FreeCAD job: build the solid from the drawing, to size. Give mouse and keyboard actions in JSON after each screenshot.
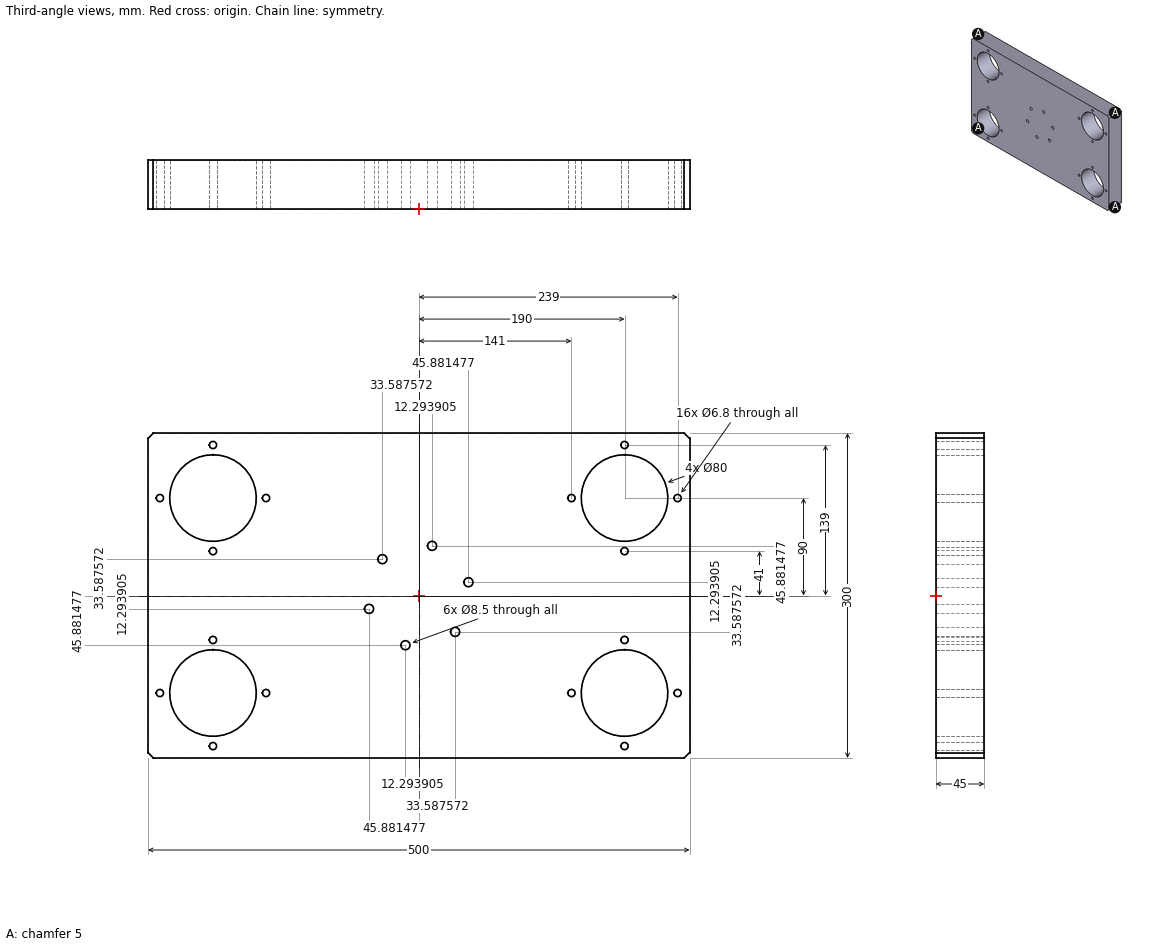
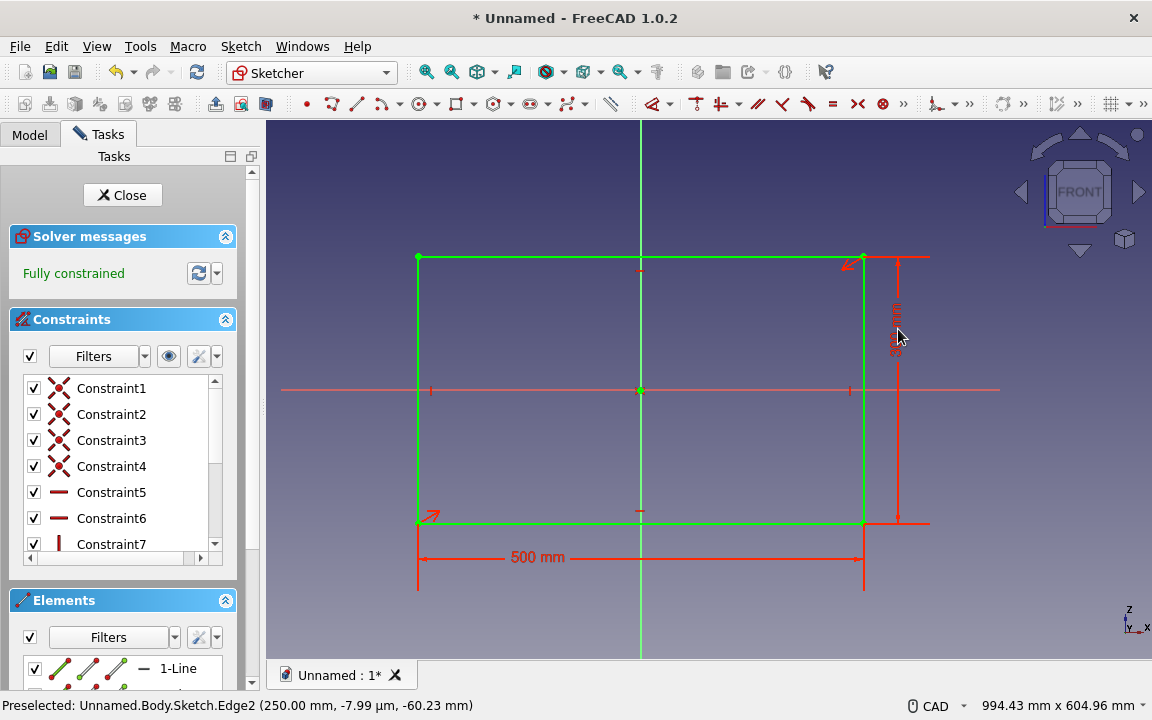
{"action": "left_click", "coordinate": [123, 195]}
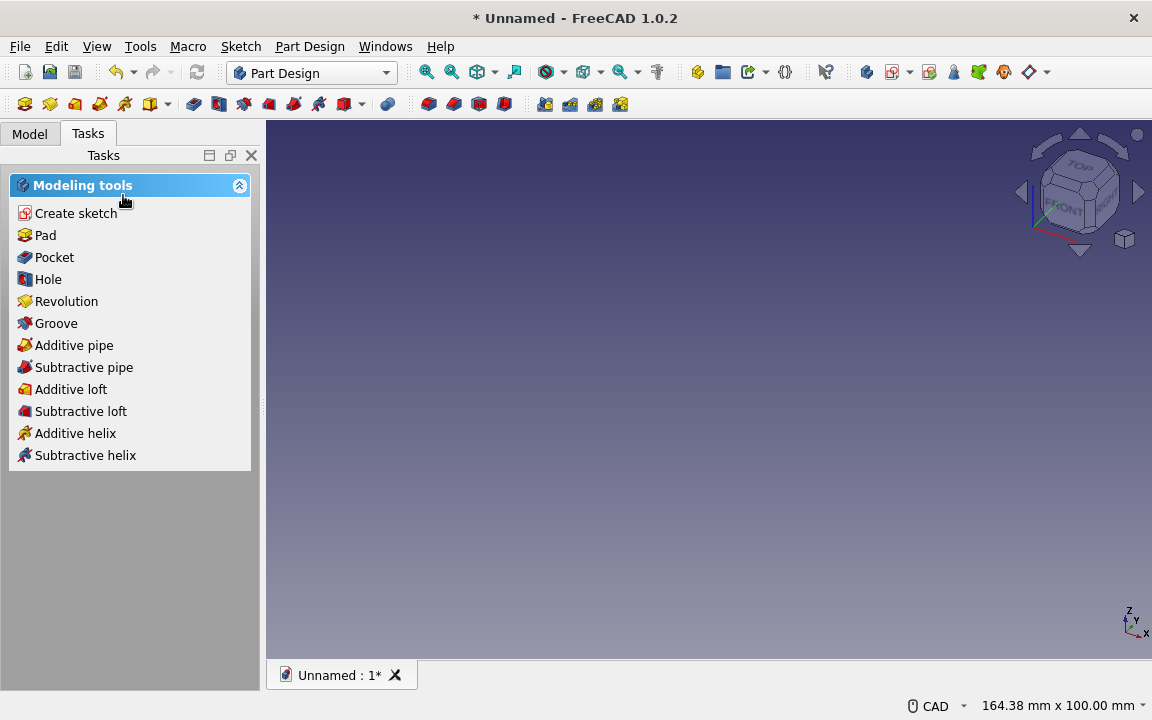
{"action": "left_click", "coordinate": [25, 104]}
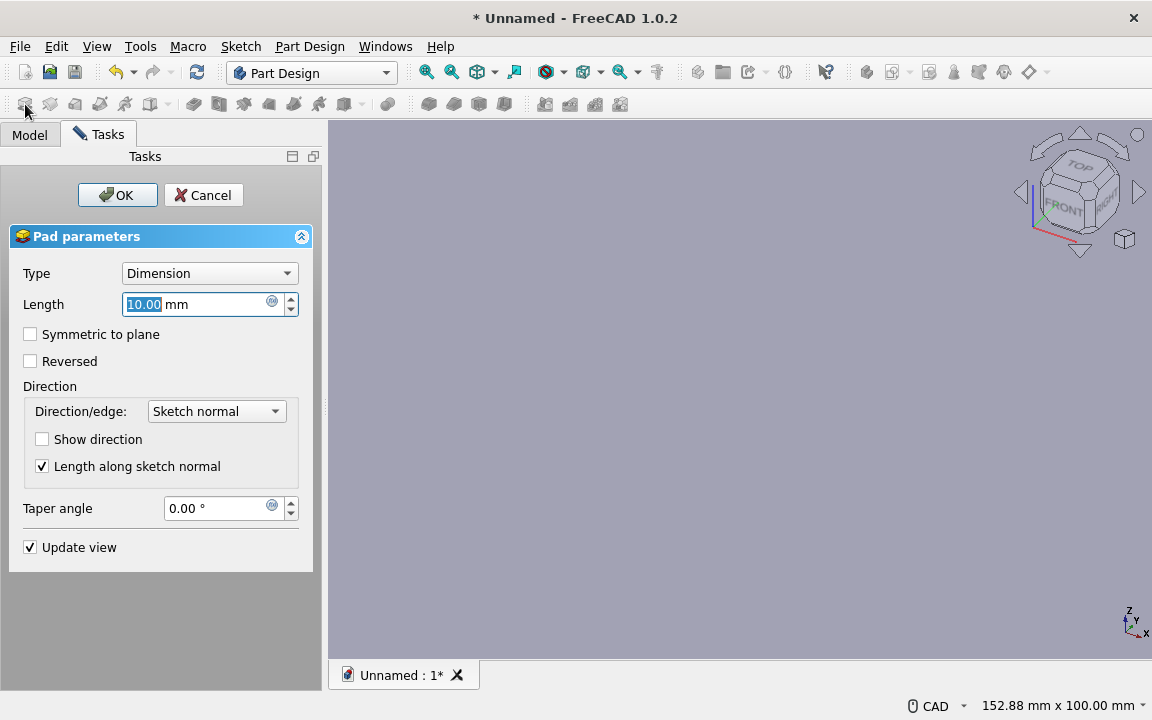
{"action": "type", "text": "45"}
{"action": "key", "text": "Tab"}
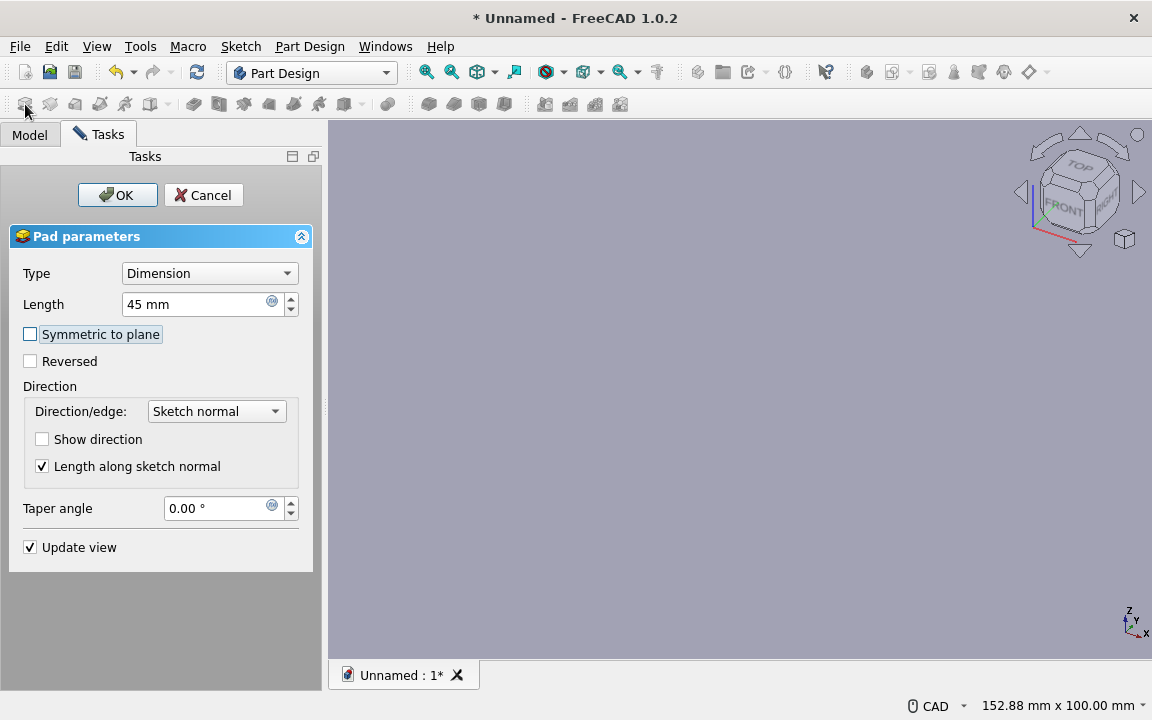
{"action": "left_click", "coordinate": [31, 361]}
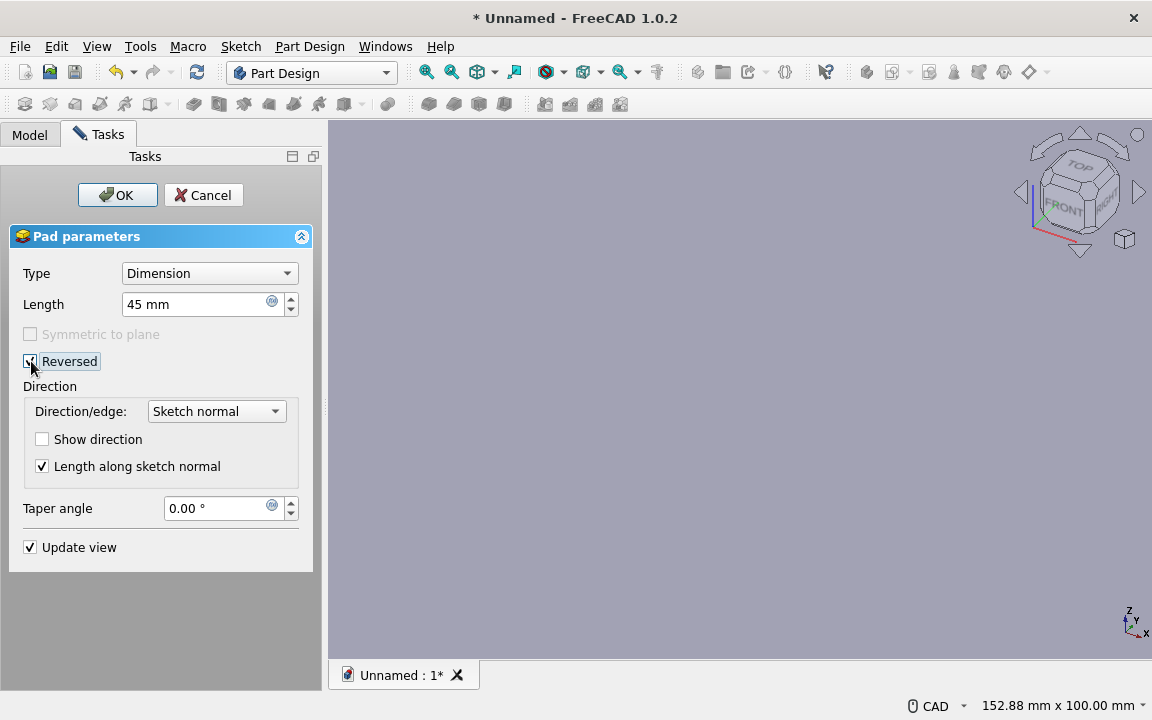
{"action": "left_click", "coordinate": [118, 195]}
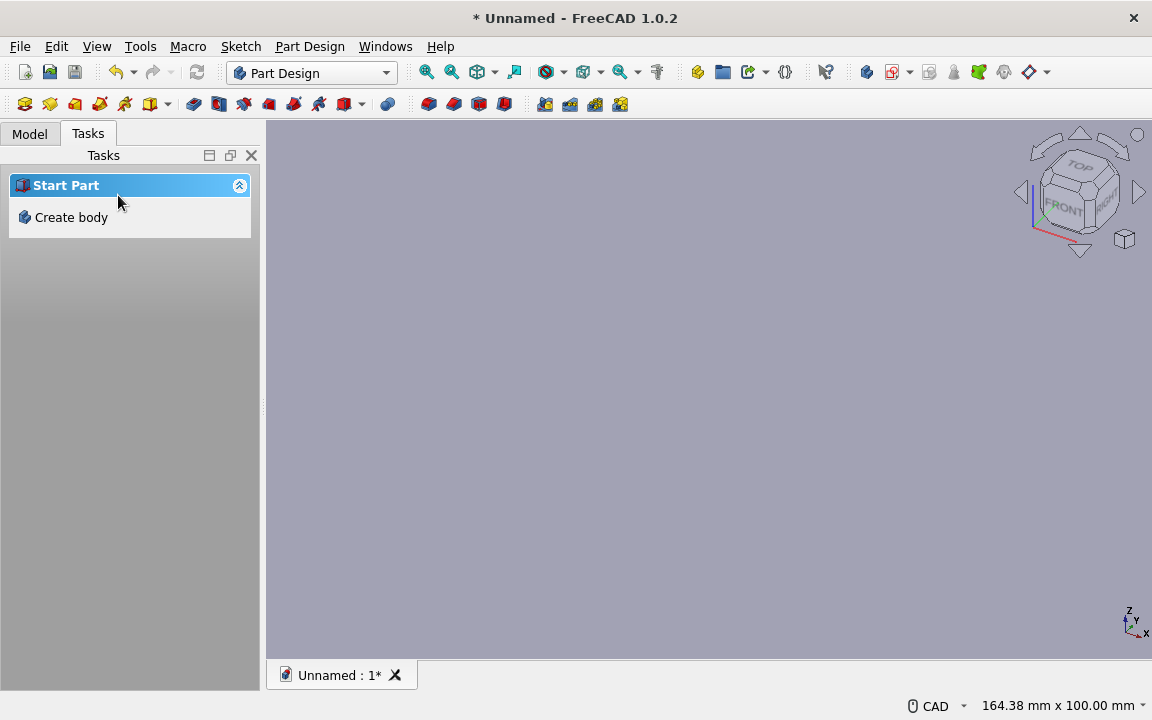
{"action": "left_click", "coordinate": [427, 72]}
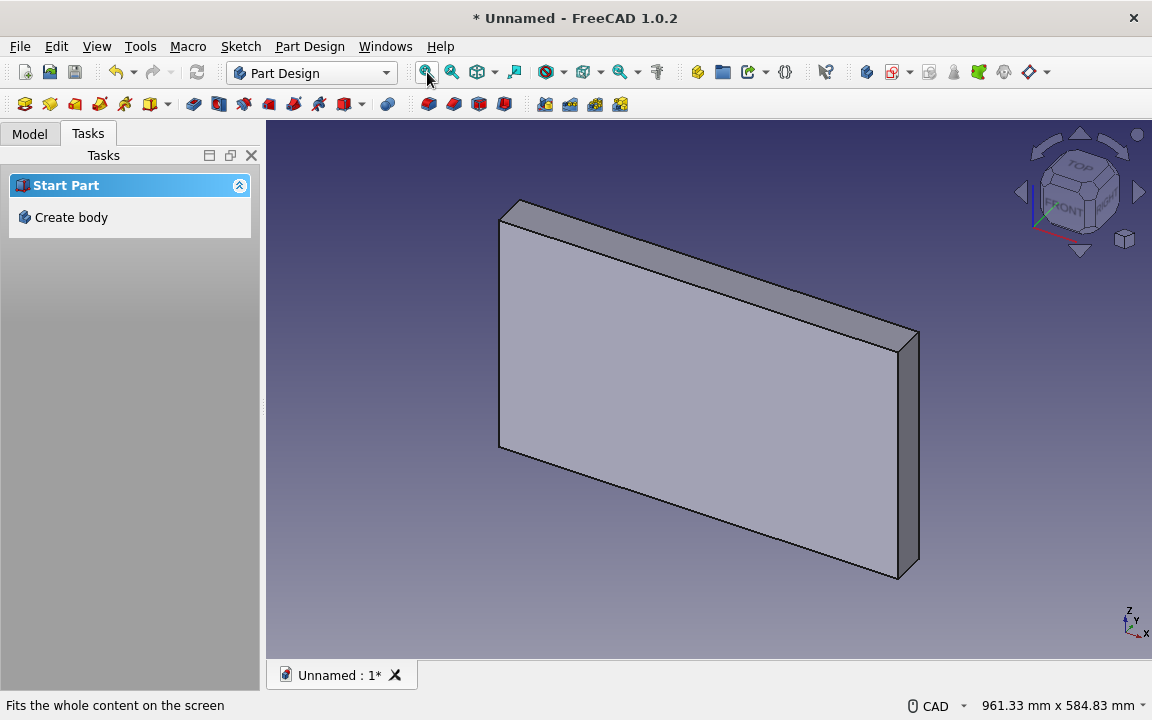
{"action": "left_click", "coordinate": [909, 341]}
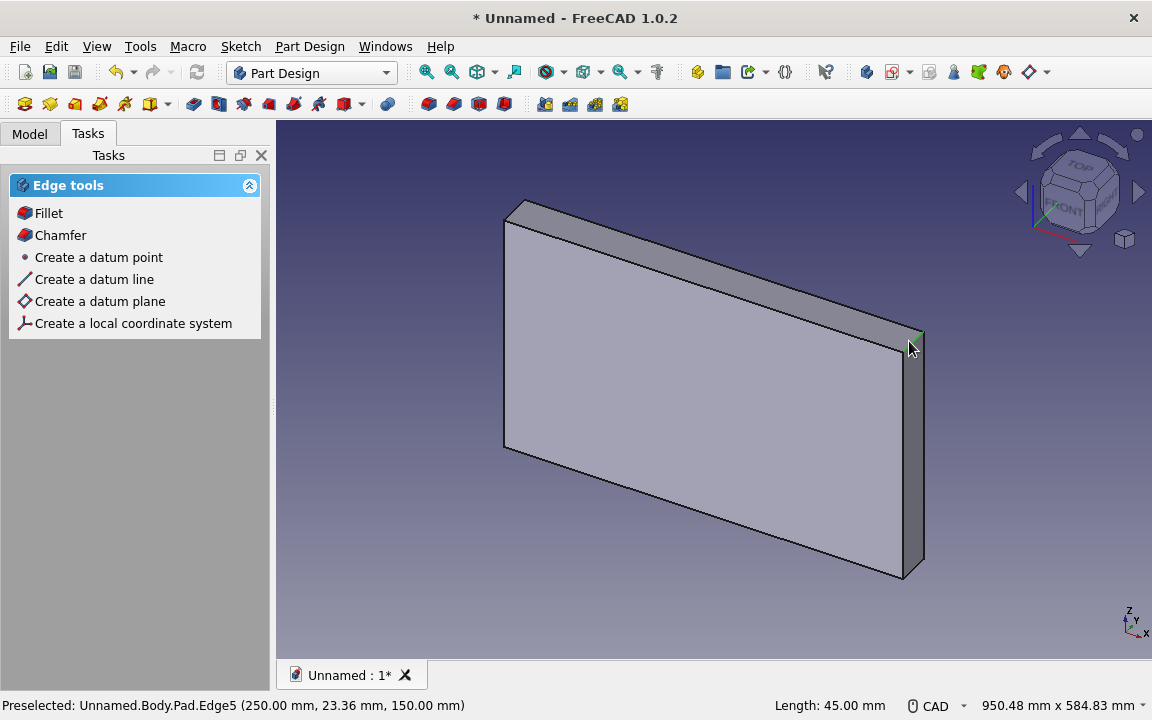
{"action": "key", "text": "0"}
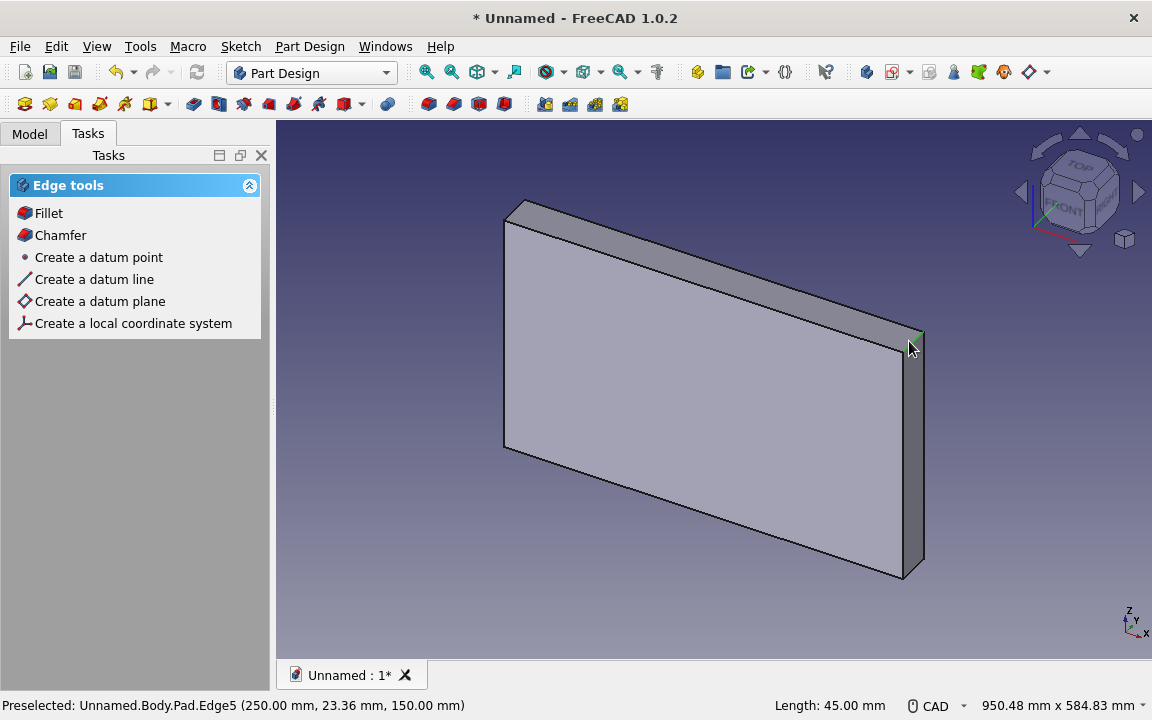
{"action": "key", "text": "2"}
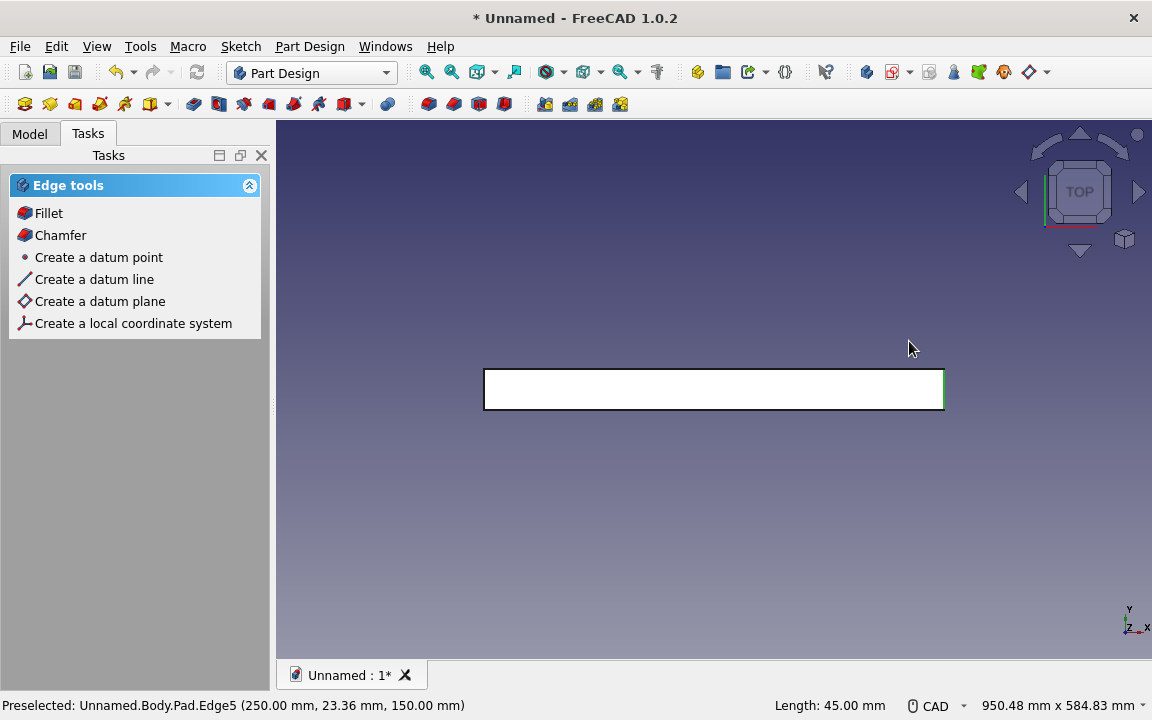
{"action": "left_click", "coordinate": [484, 388], "text": "ctrl"}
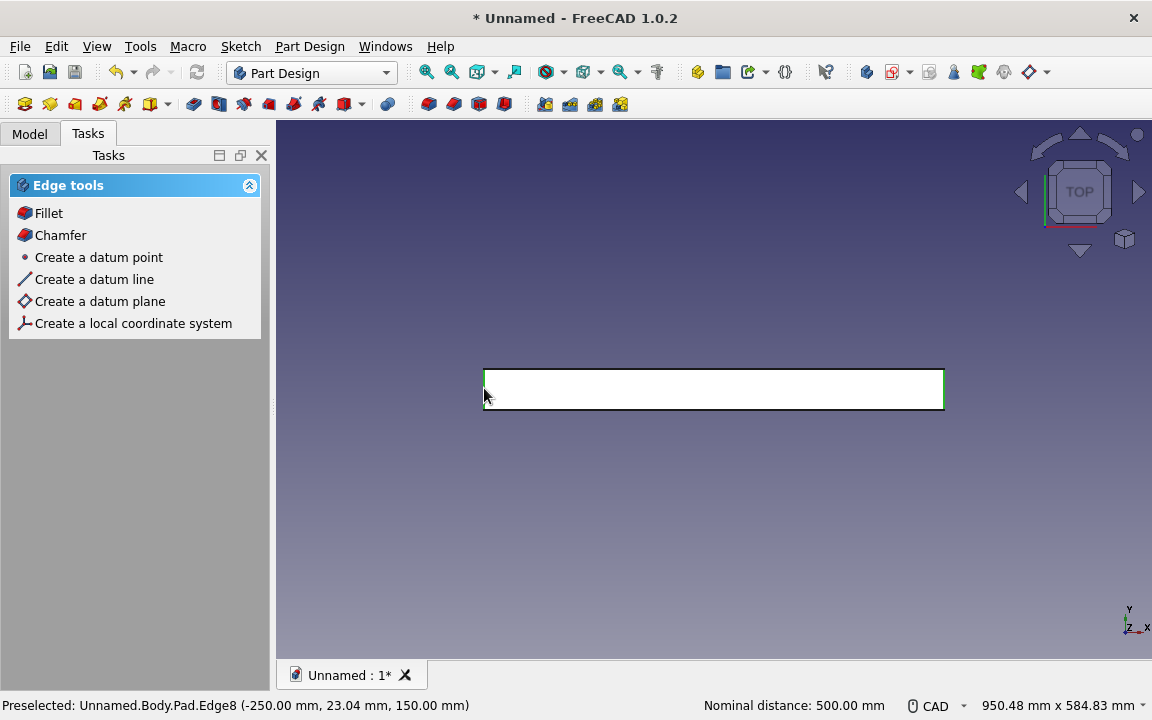
{"action": "key", "text": "1"}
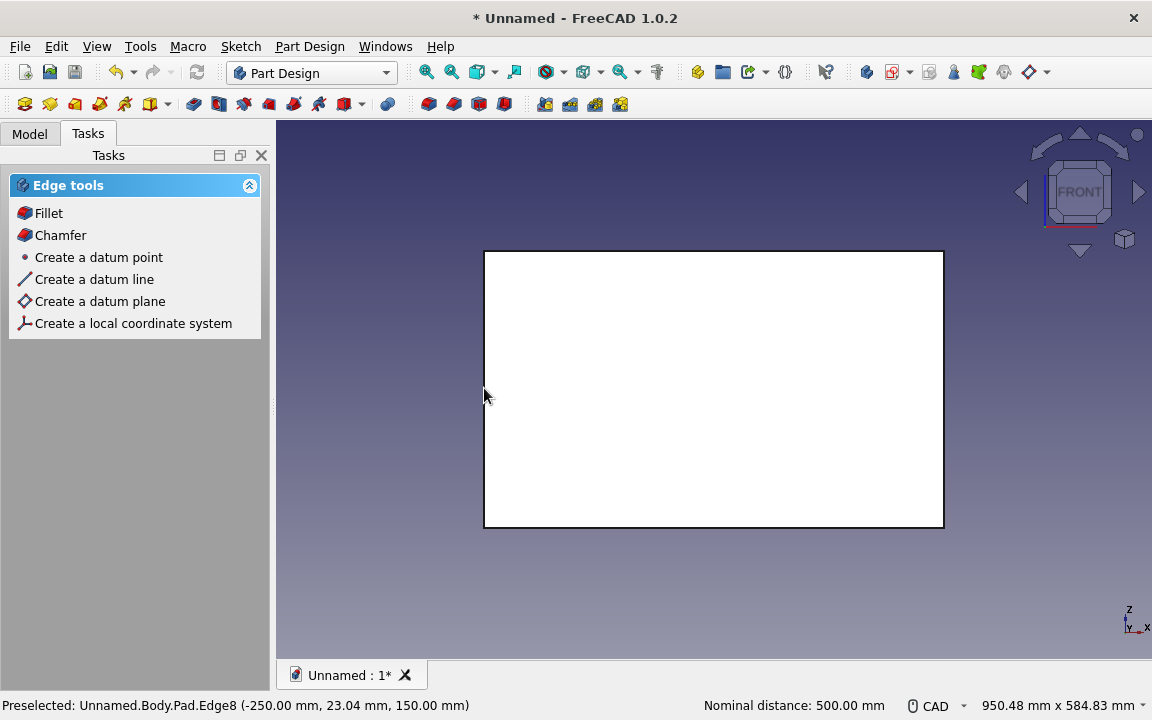
{"action": "key", "text": "3"}